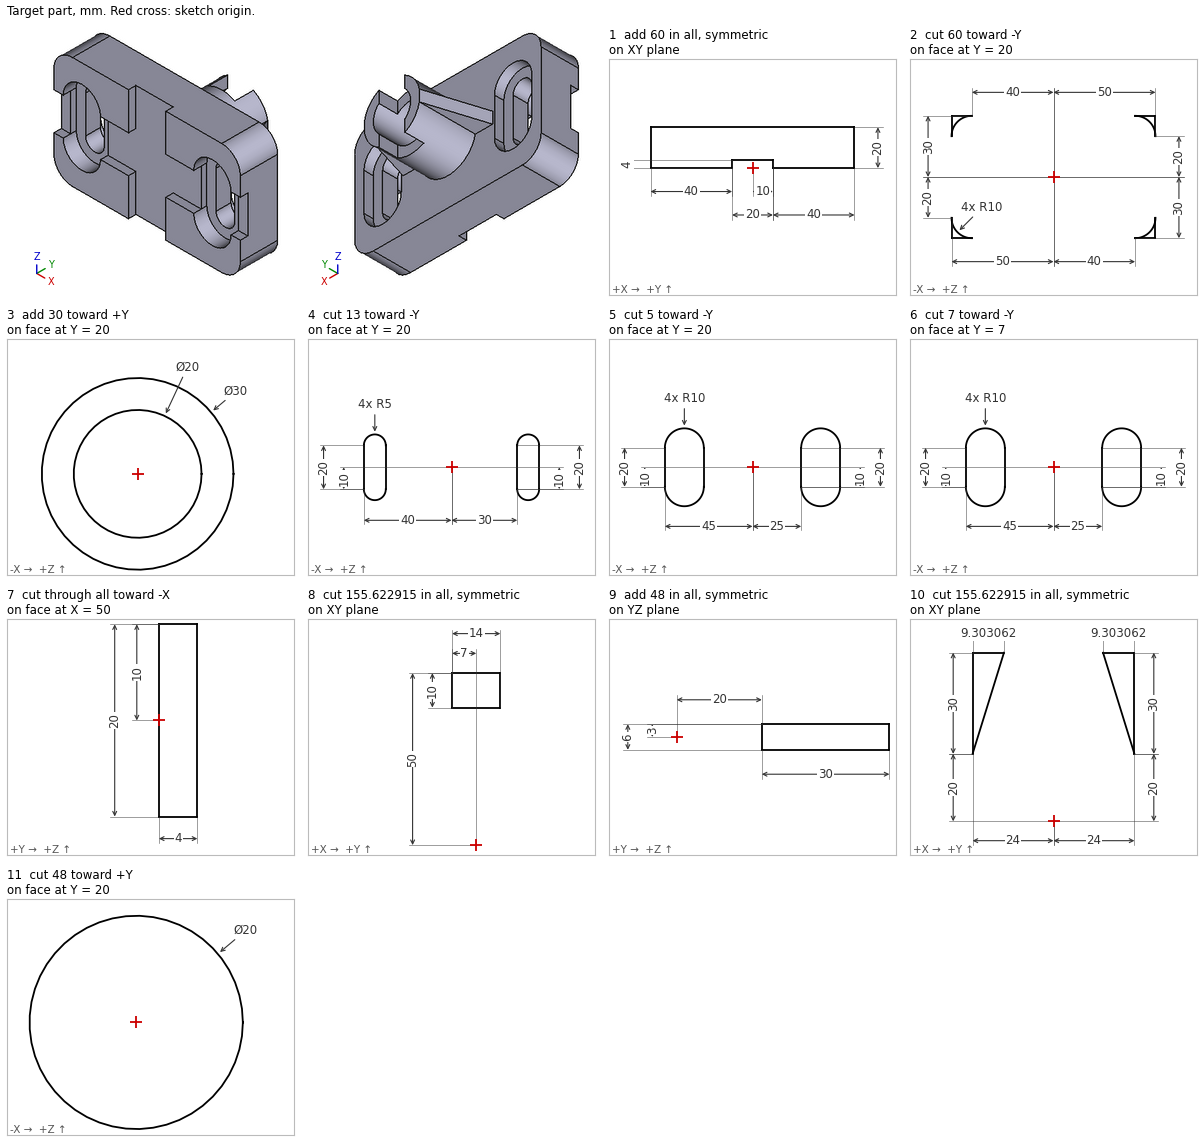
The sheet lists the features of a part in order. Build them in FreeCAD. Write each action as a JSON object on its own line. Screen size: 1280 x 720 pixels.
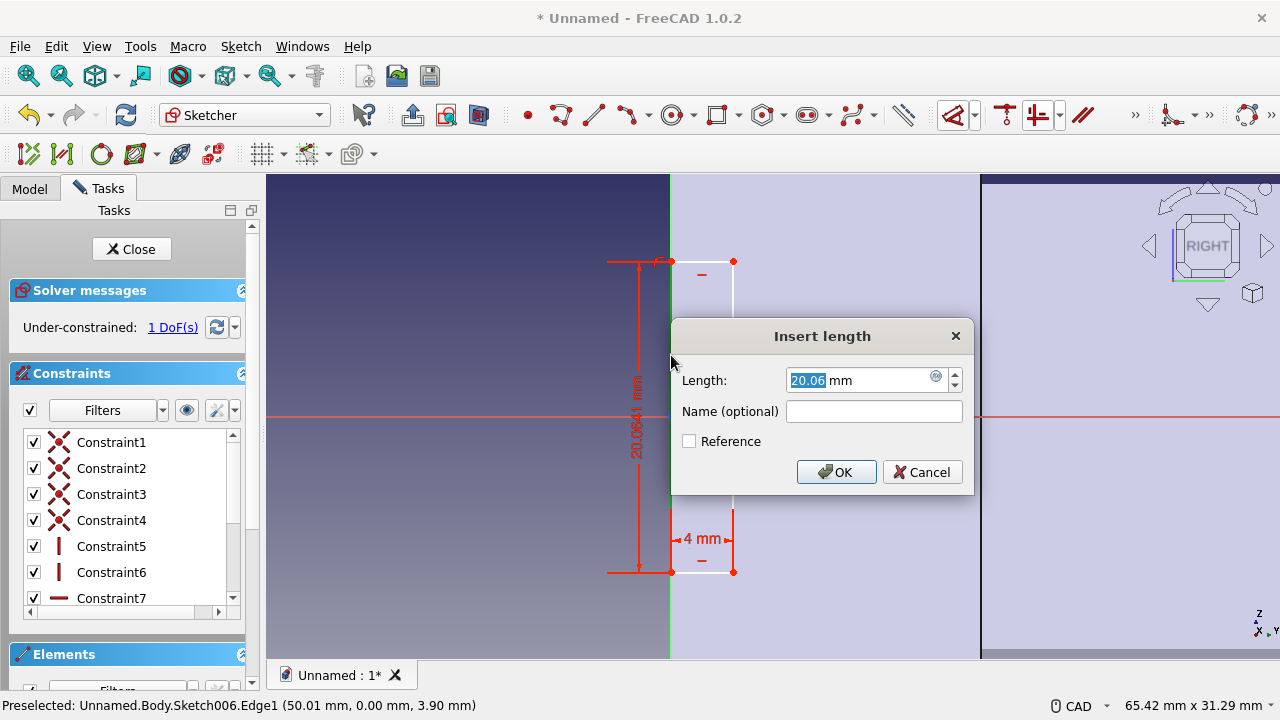
{"action": "type", "text": "20"}
{"action": "key", "text": "Return"}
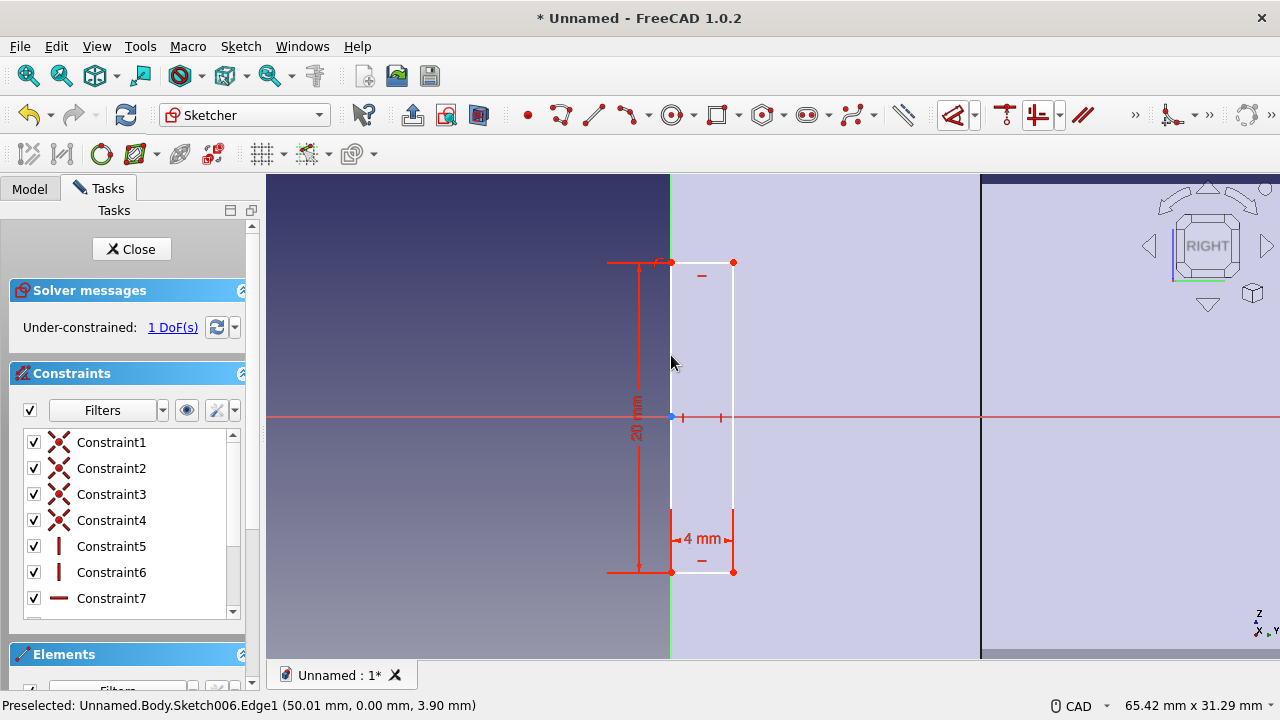
{"action": "left_click", "coordinate": [671, 263]}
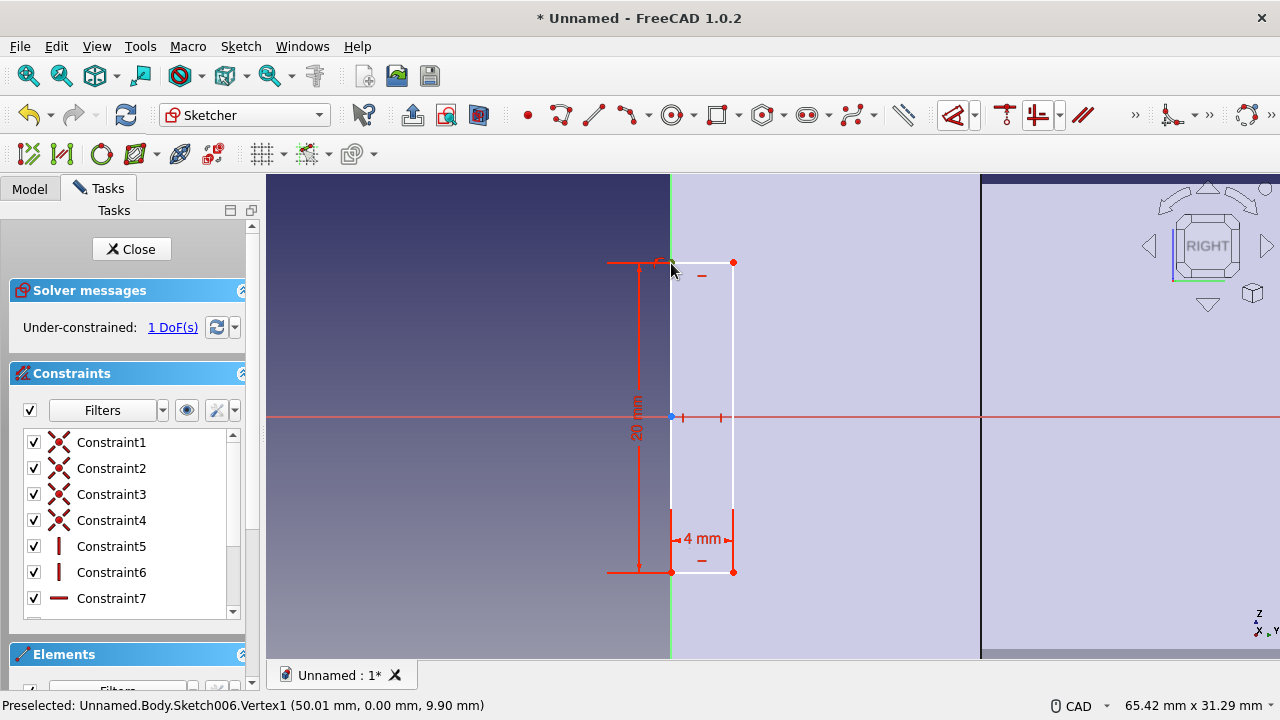
{"action": "key", "text": "i"}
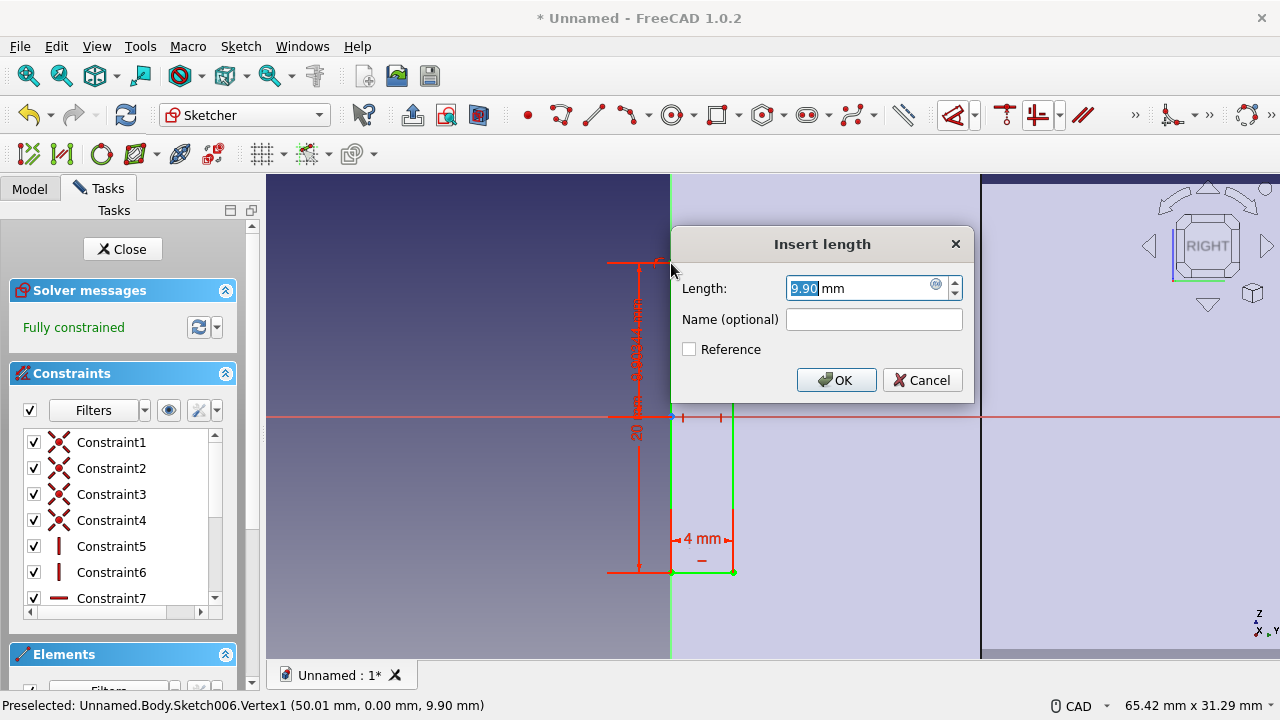
{"action": "type", "text": "10"}
{"action": "key", "text": "Return"}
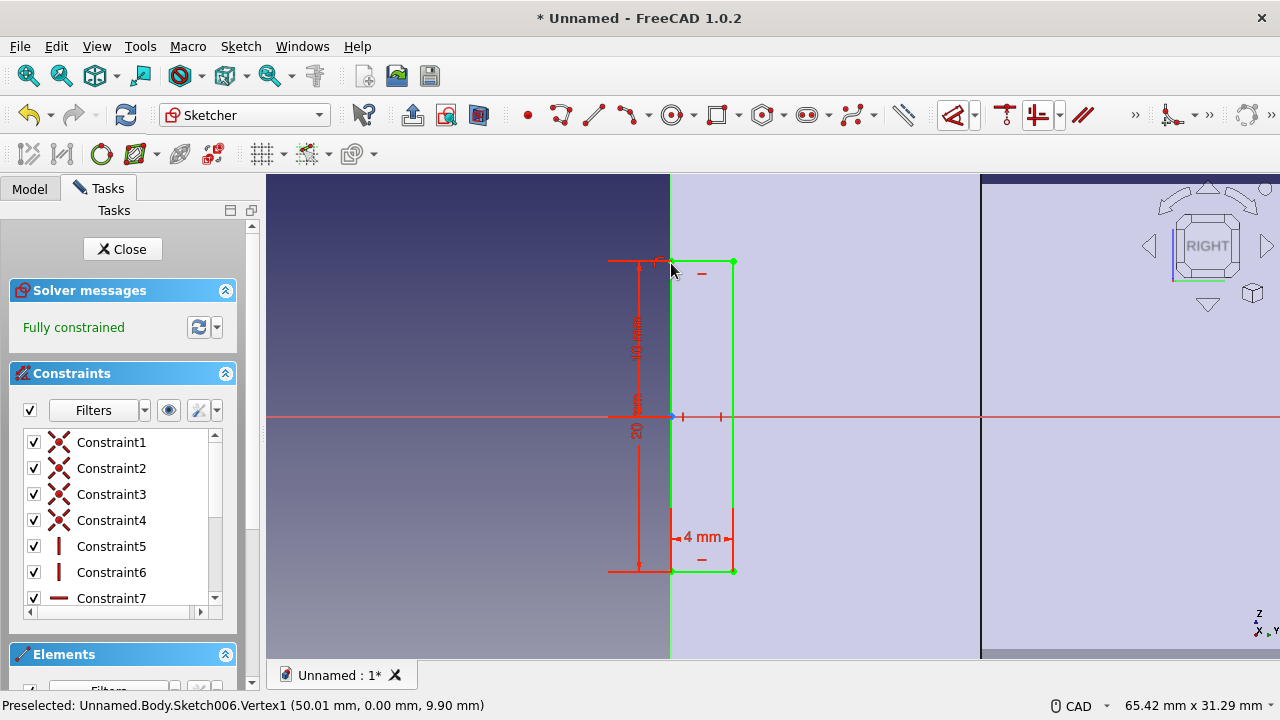
{"action": "left_click", "coordinate": [123, 249]}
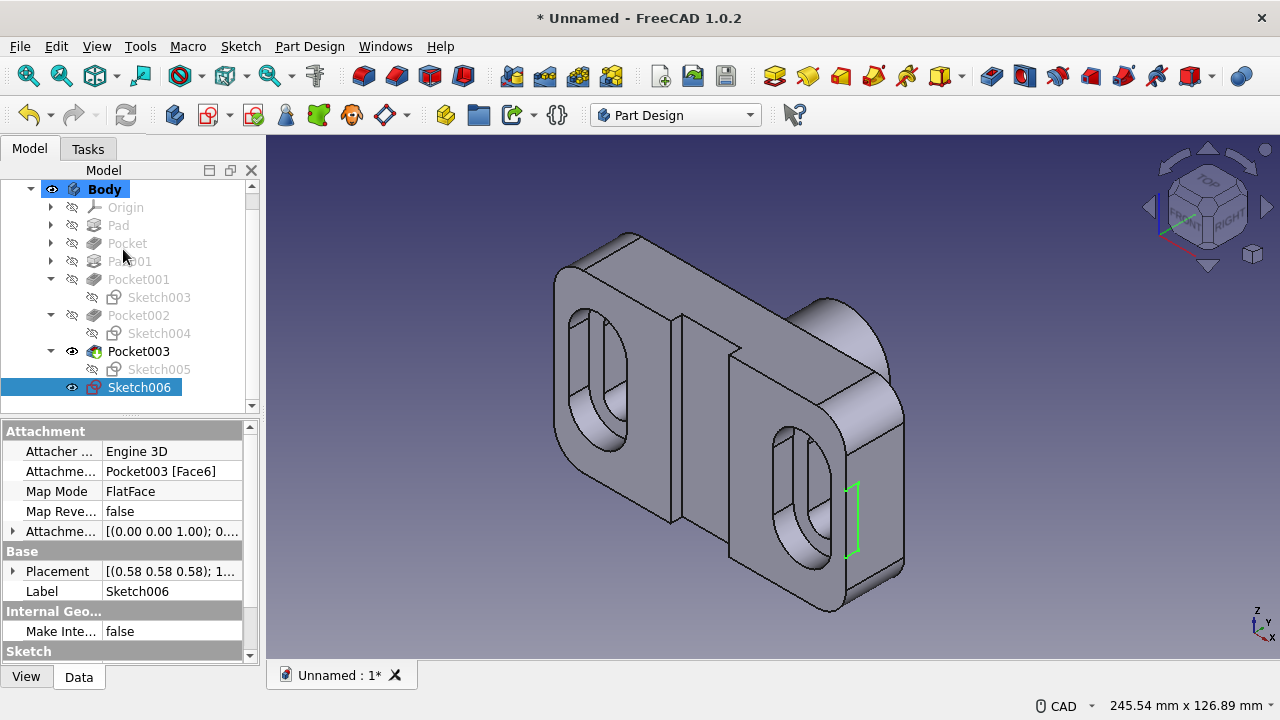
{"action": "left_click", "coordinate": [992, 76]}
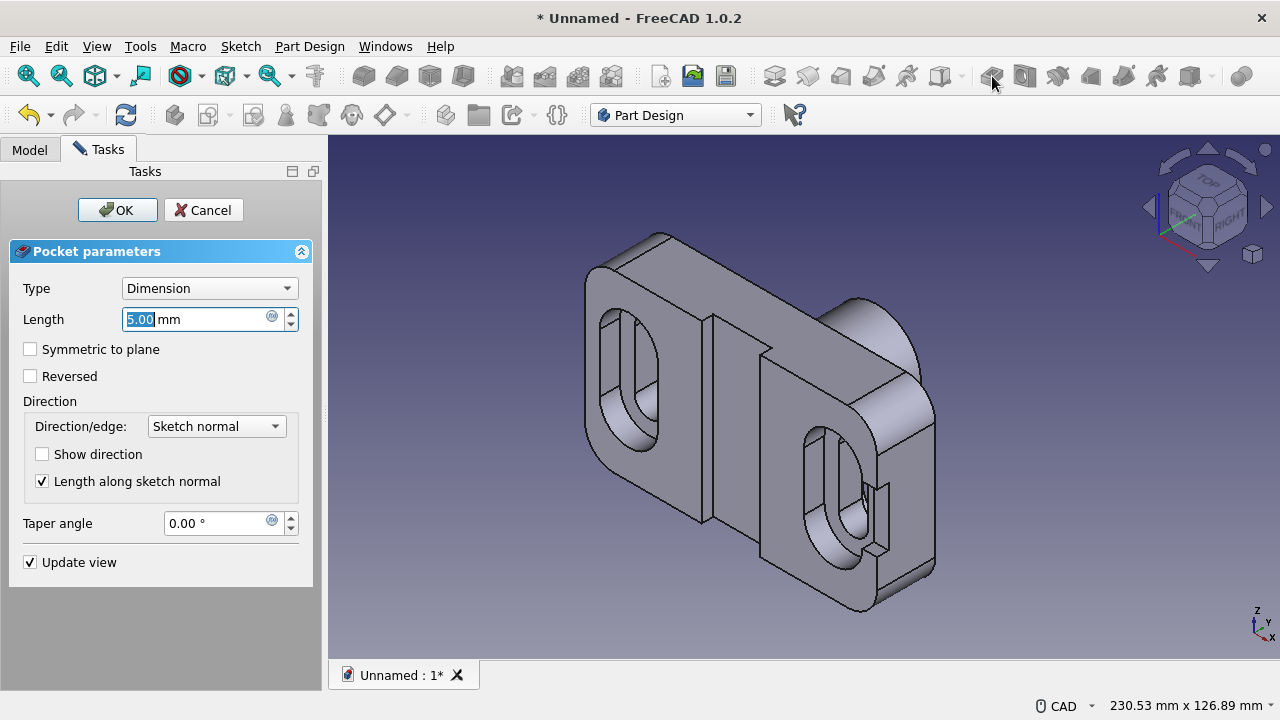
{"action": "left_click", "coordinate": [210, 288]}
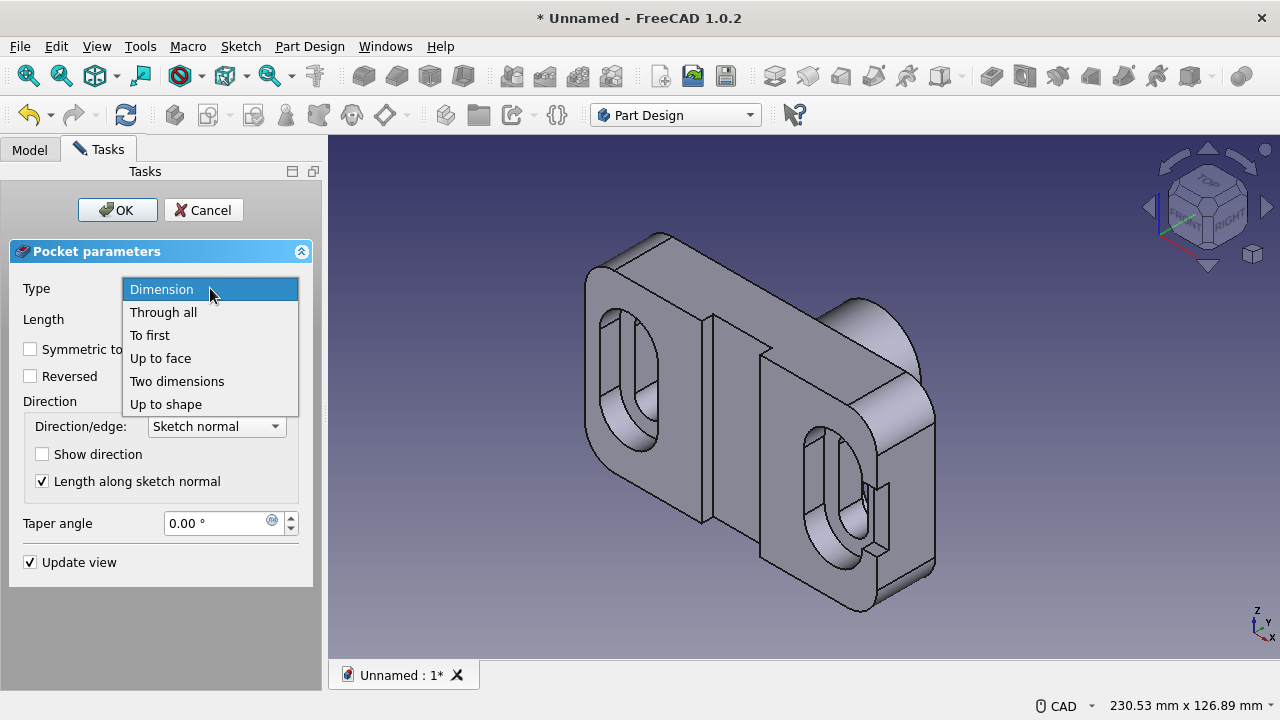
{"action": "left_click", "coordinate": [208, 312]}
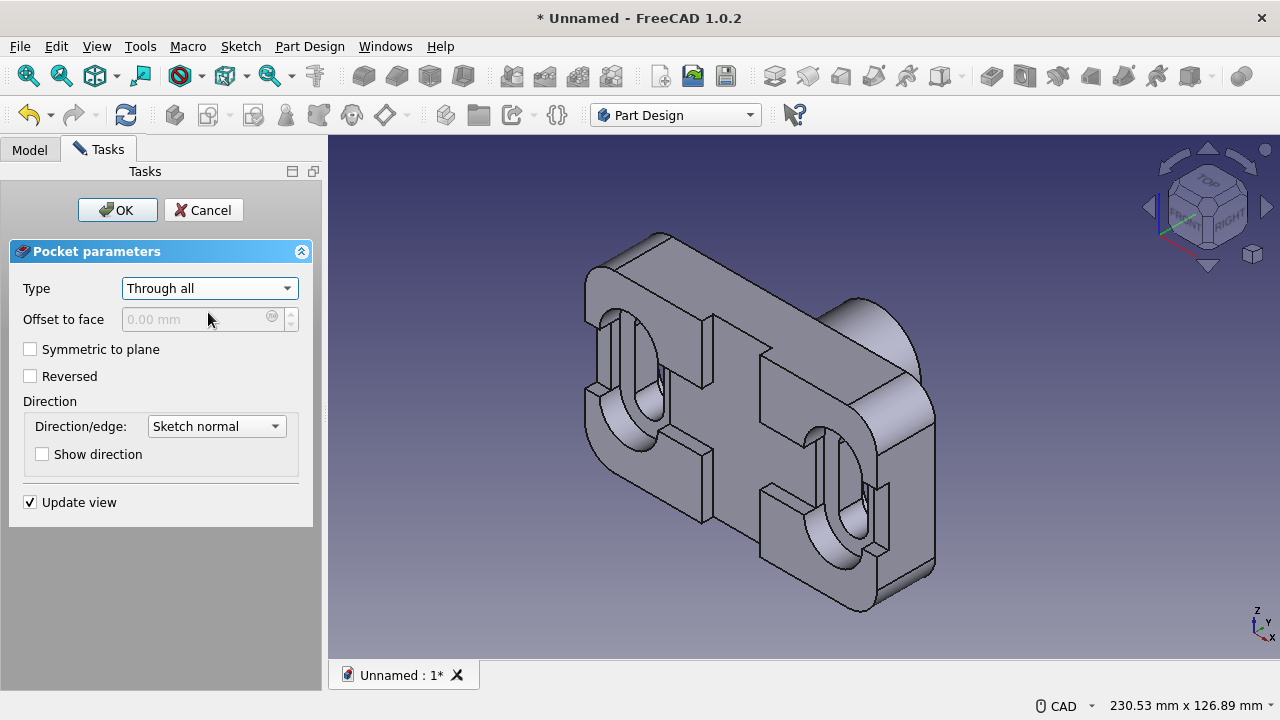
{"action": "left_click", "coordinate": [118, 210]}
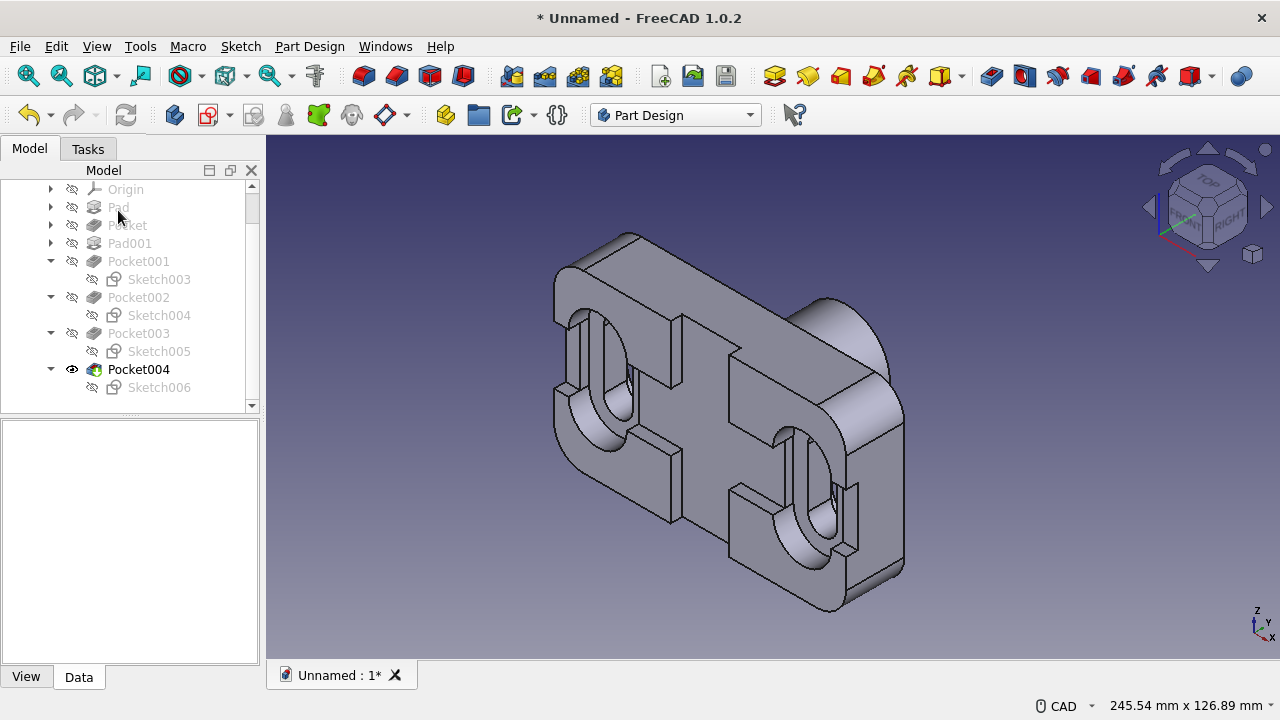
{"action": "left_click", "coordinate": [208, 116]}